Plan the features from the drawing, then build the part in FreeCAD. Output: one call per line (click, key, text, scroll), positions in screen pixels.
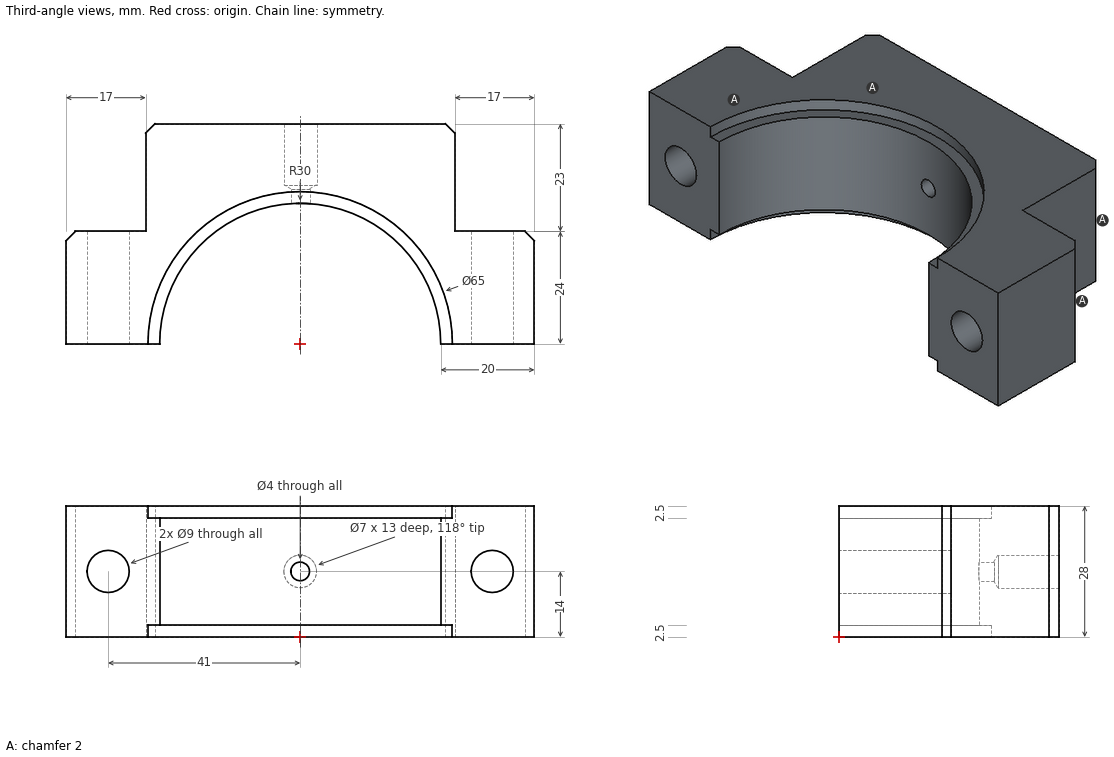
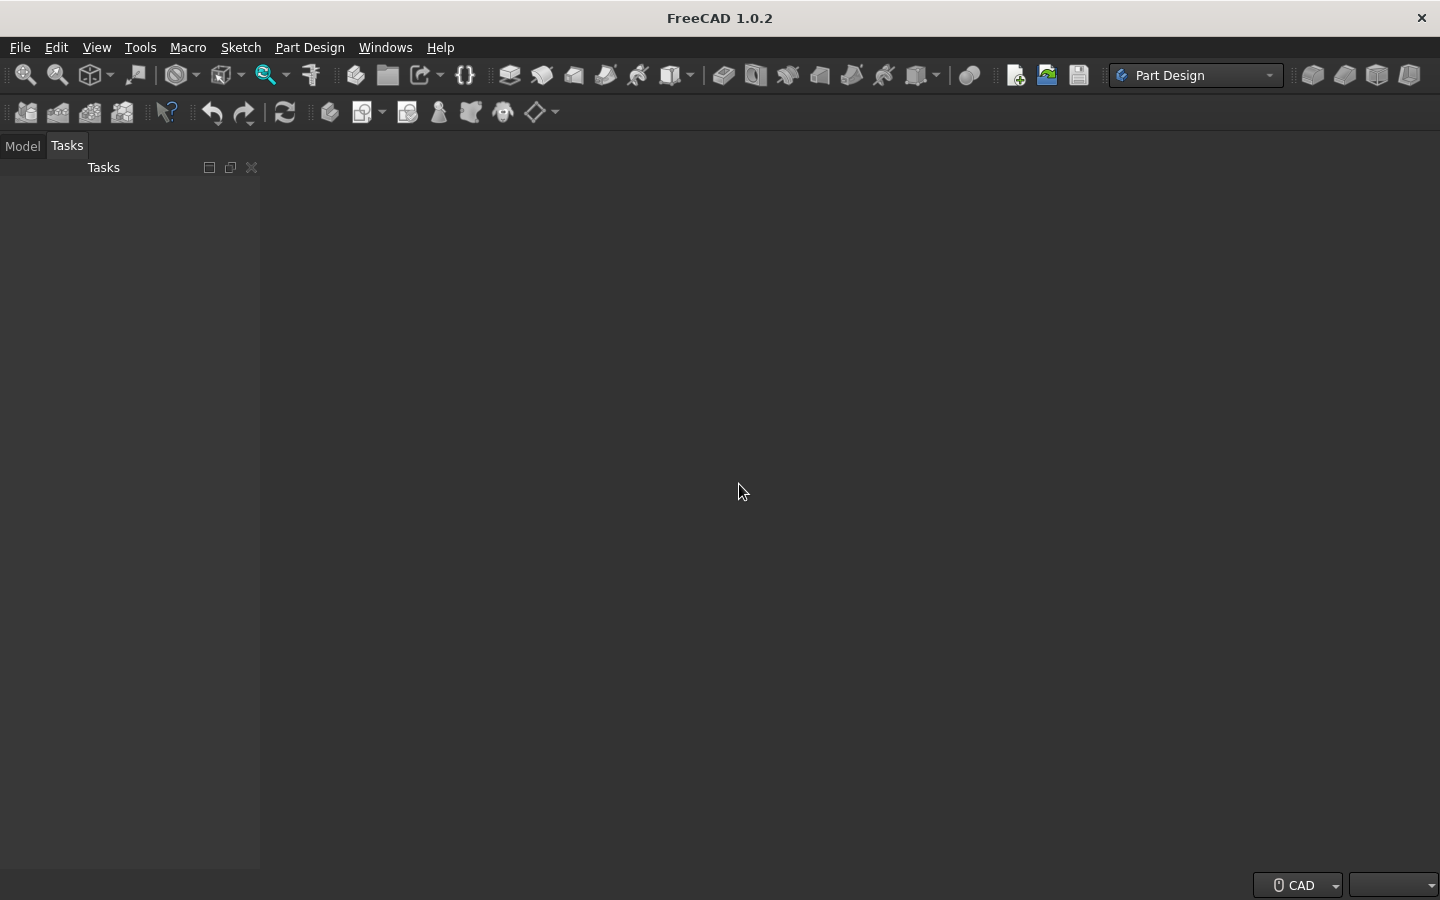
click(1016, 76)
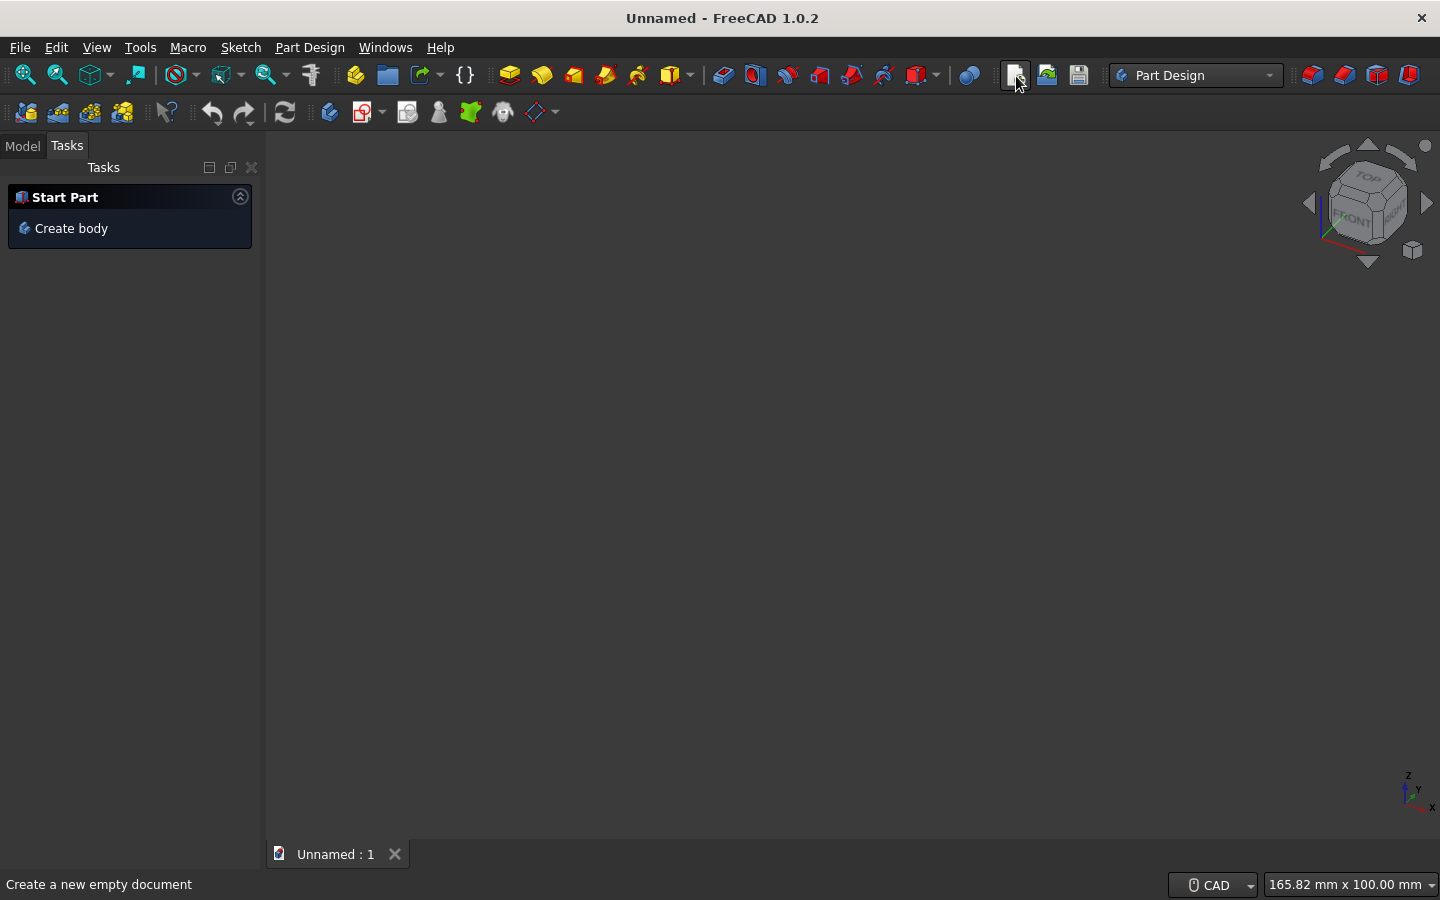
click(362, 112)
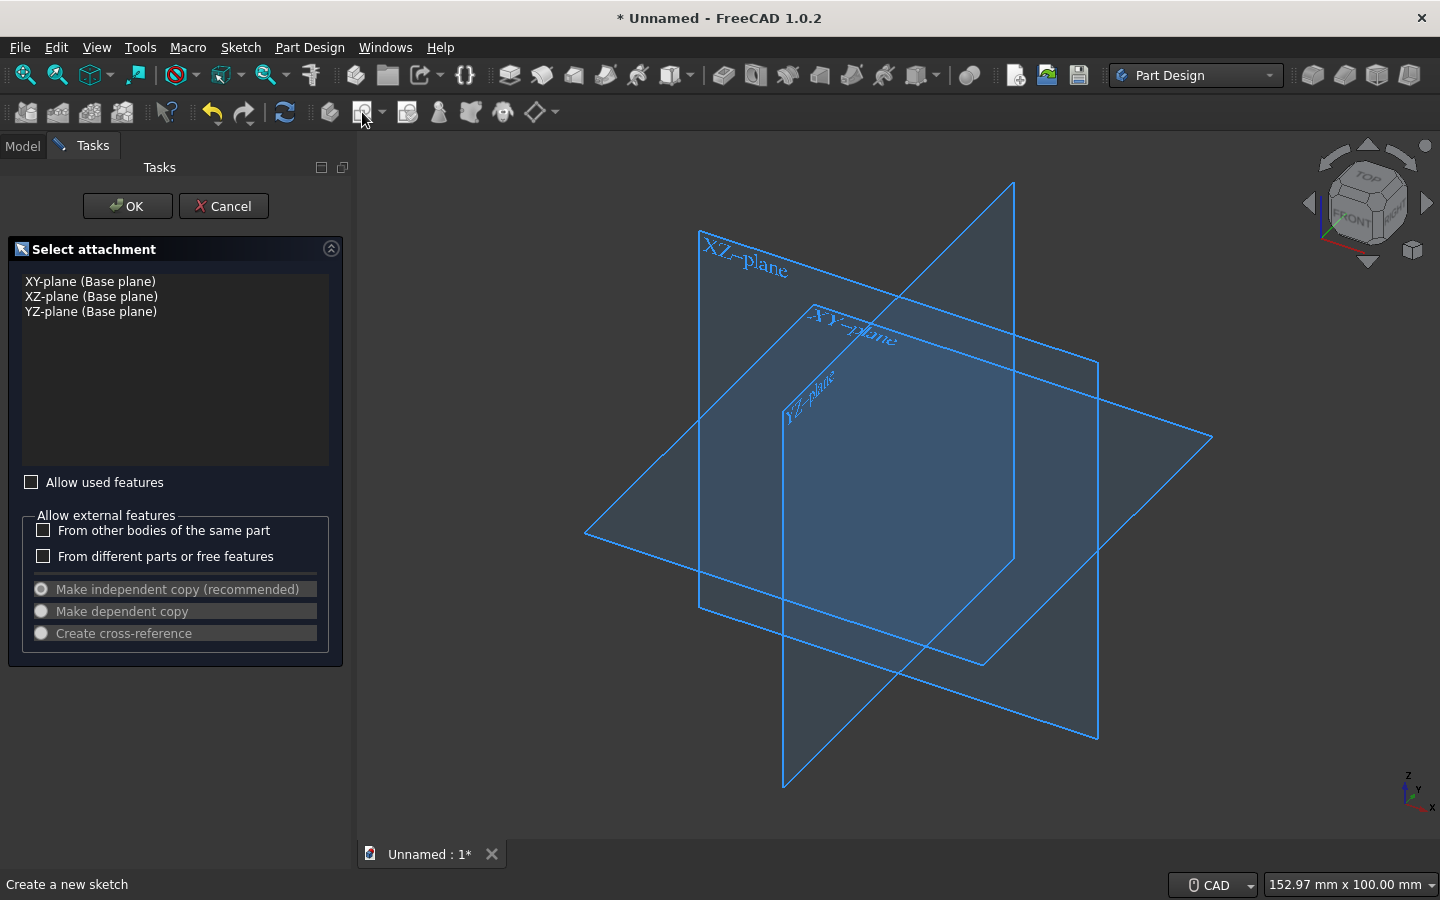
click(82, 282)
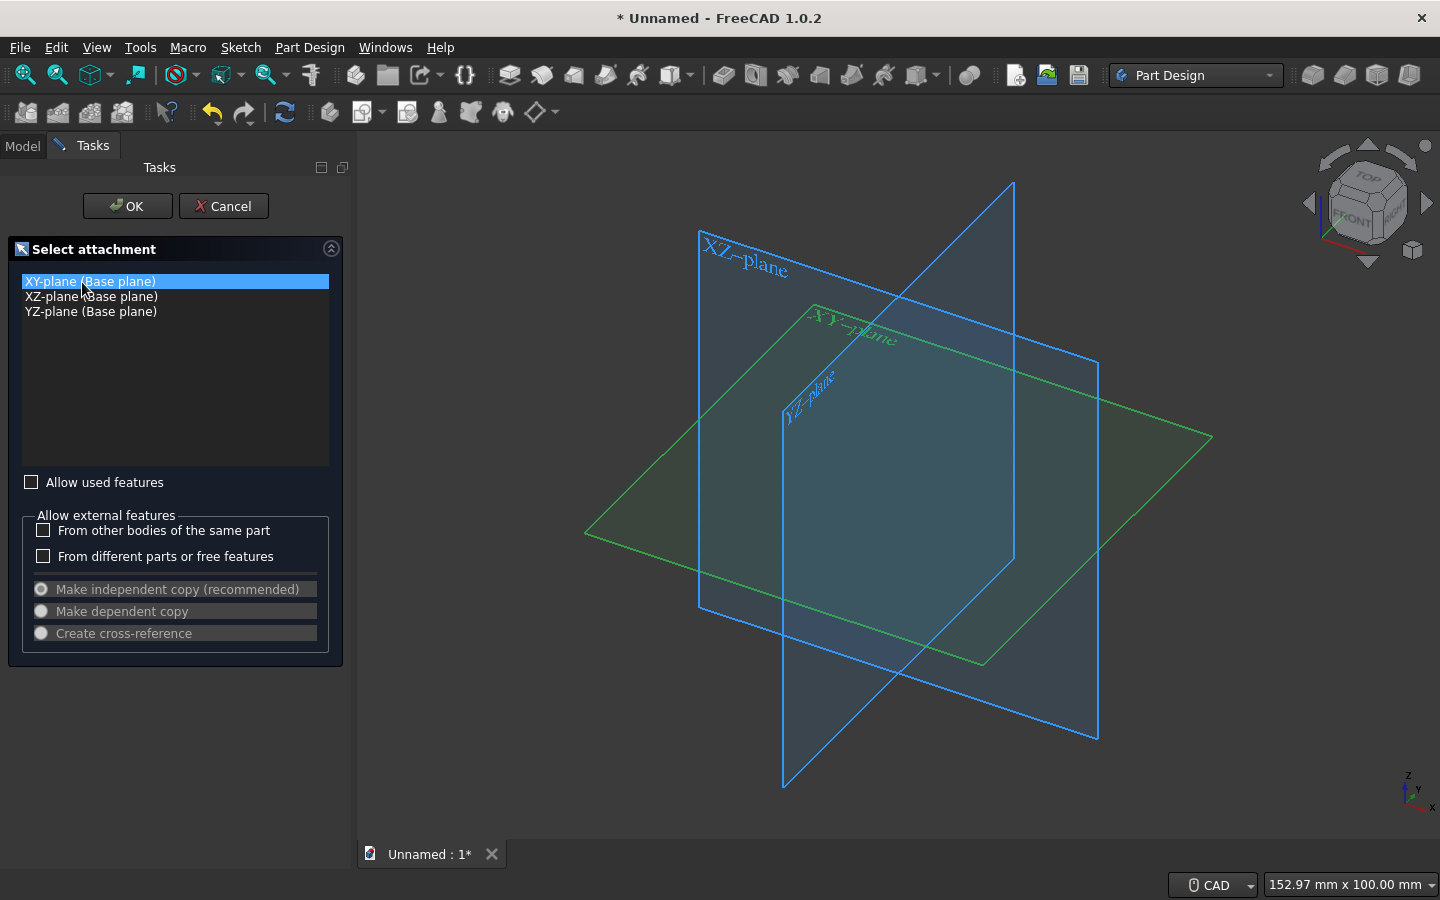
click(128, 206)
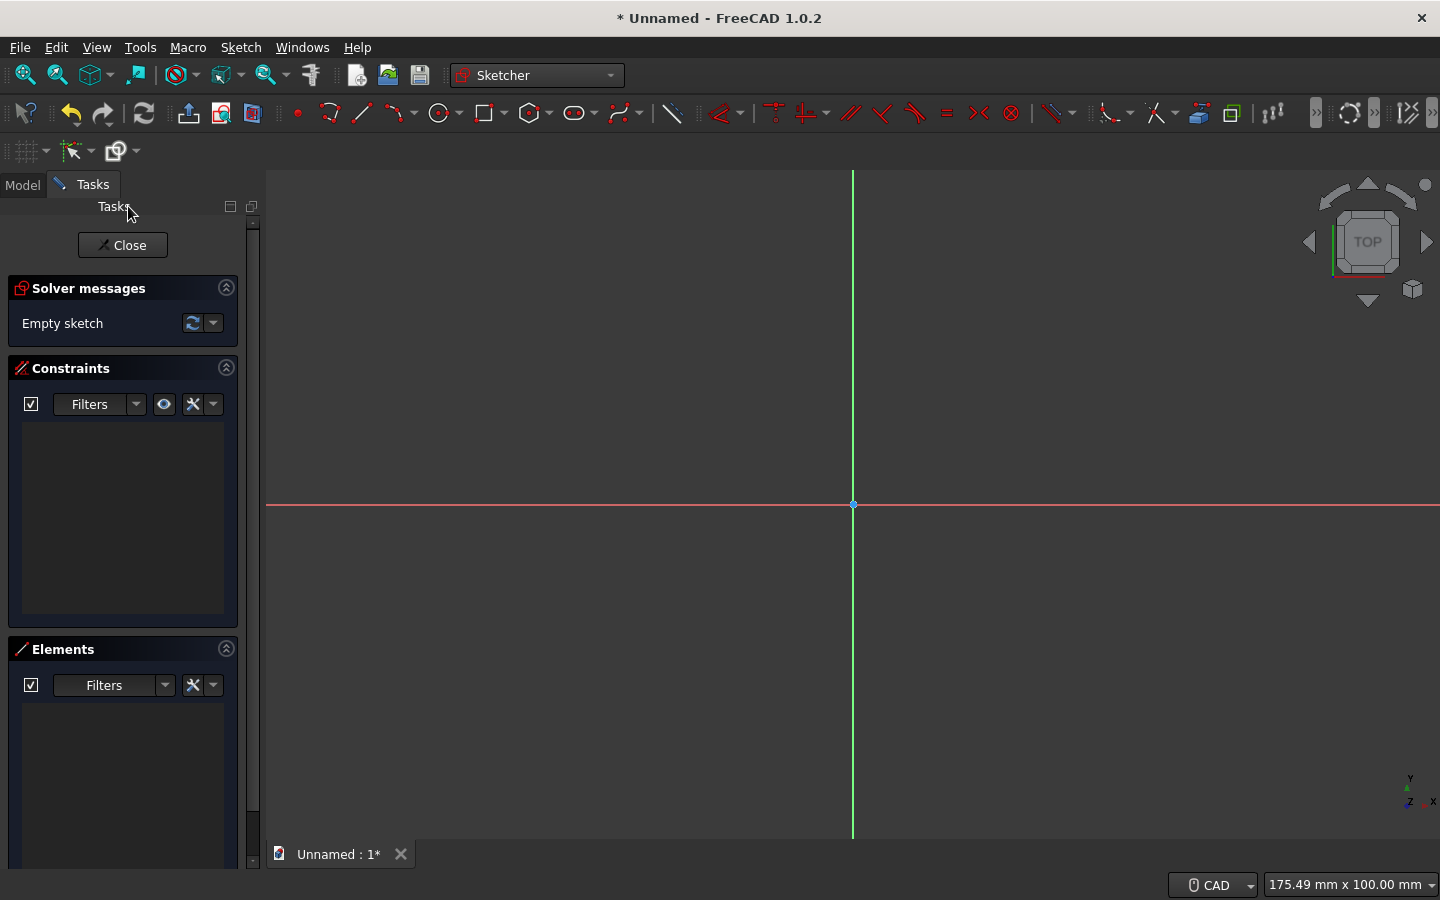
scroll(475, 811, down, 1)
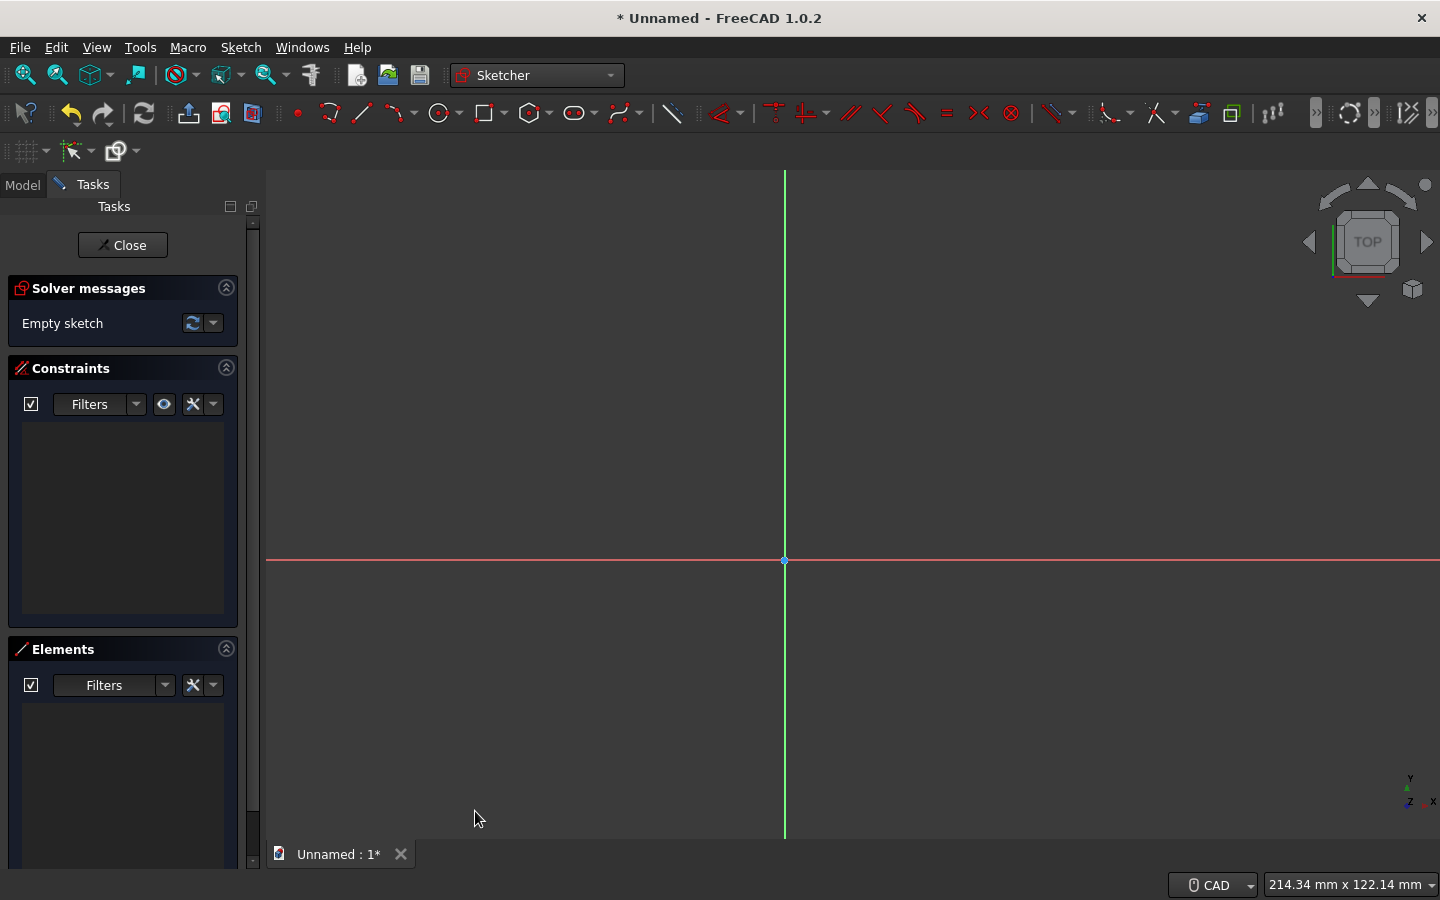
click(330, 114)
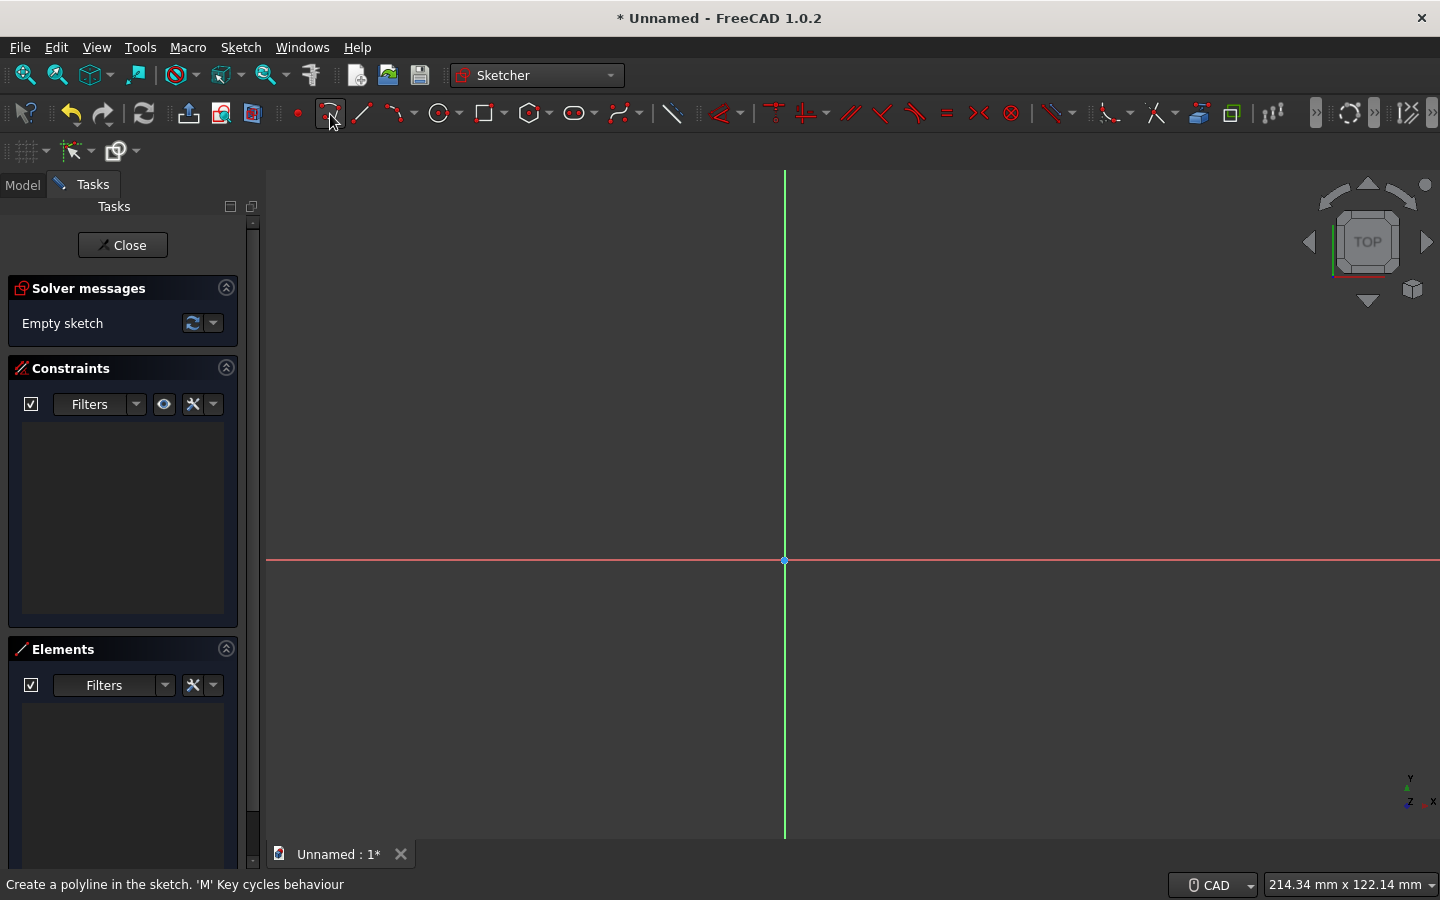
click(949, 560)
click(1058, 551)
click(1058, 429)
click(965, 429)
click(965, 303)
click(604, 303)
click(604, 429)
click(511, 429)
click(511, 560)
click(620, 551)
right_click(620, 551)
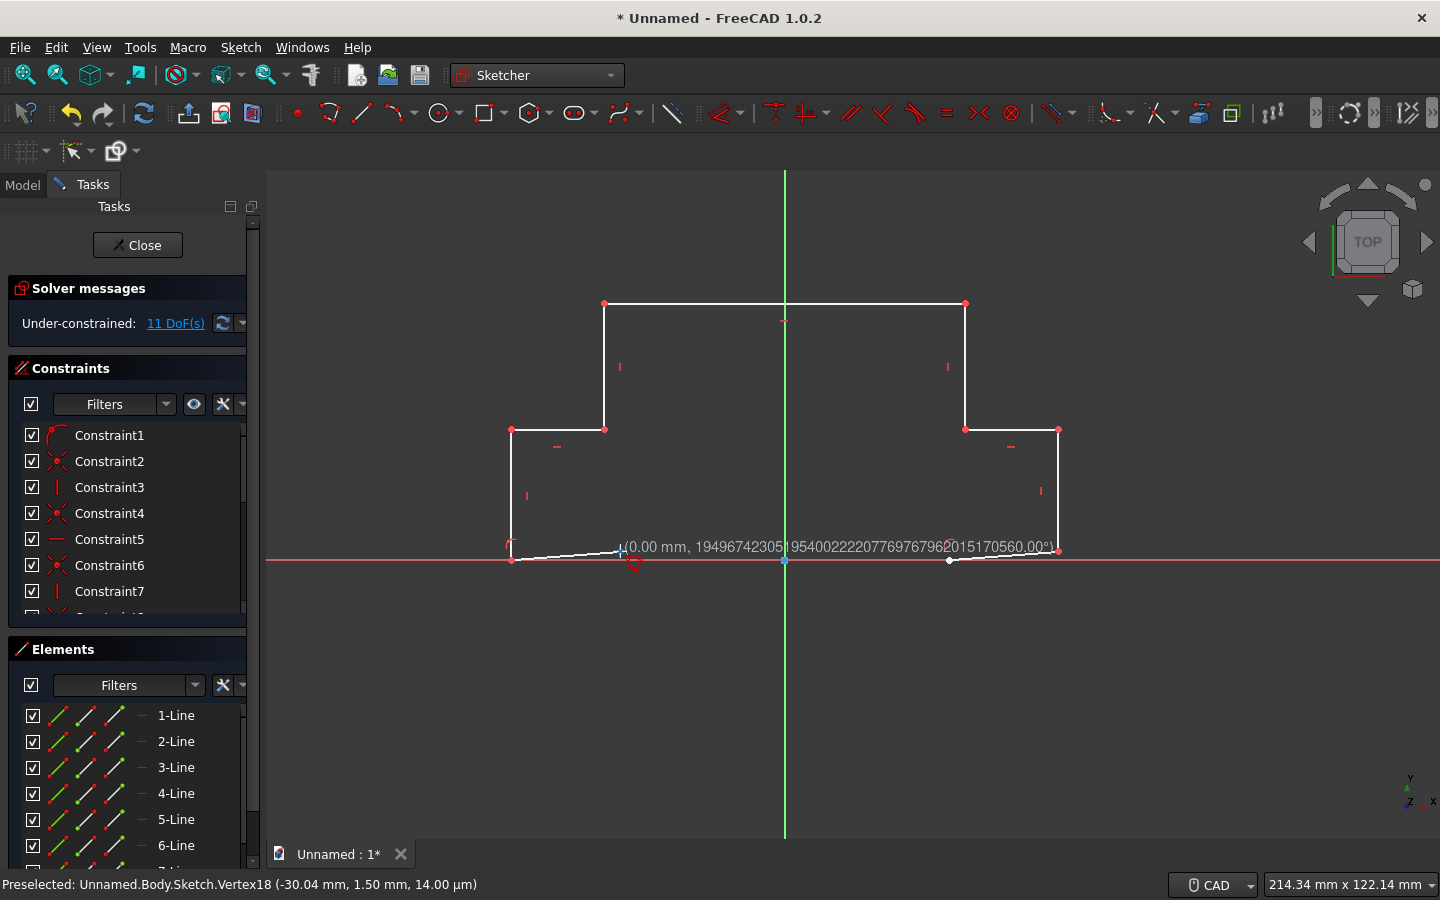
click(394, 114)